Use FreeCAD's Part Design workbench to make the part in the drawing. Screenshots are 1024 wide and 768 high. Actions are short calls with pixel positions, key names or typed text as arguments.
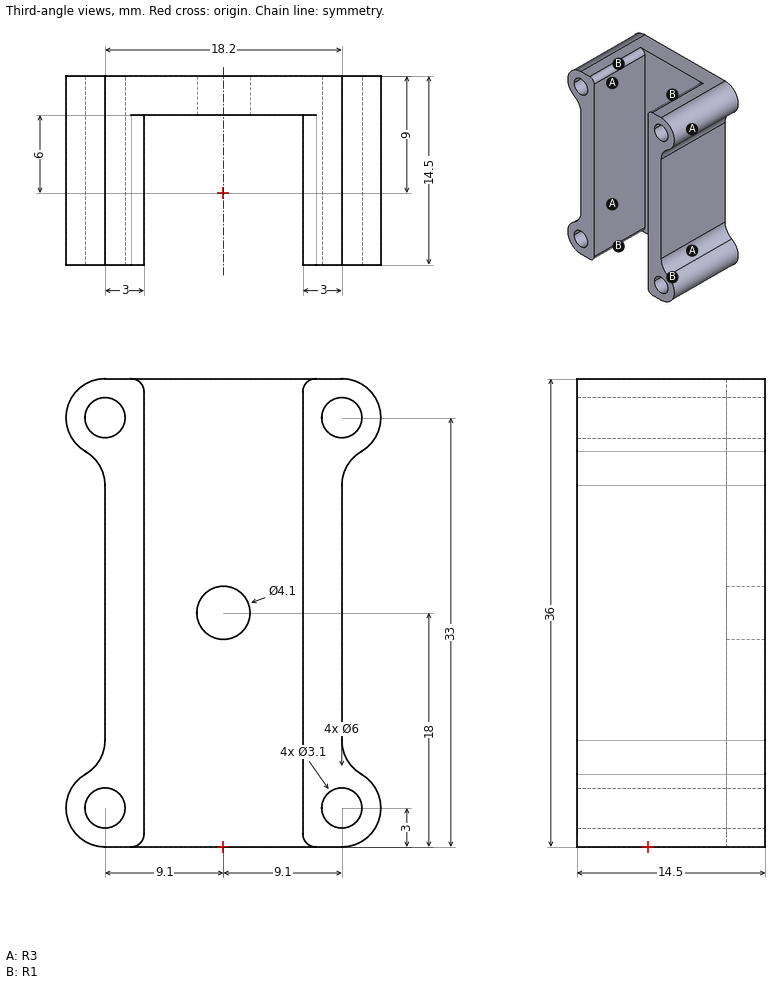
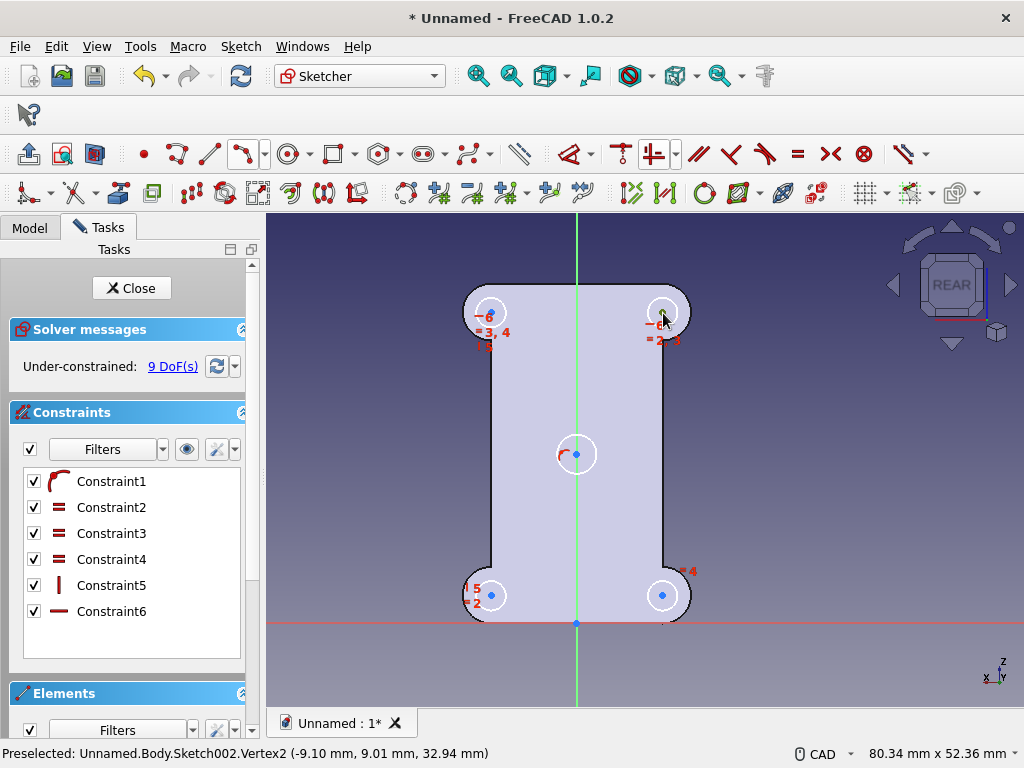
click(663, 596)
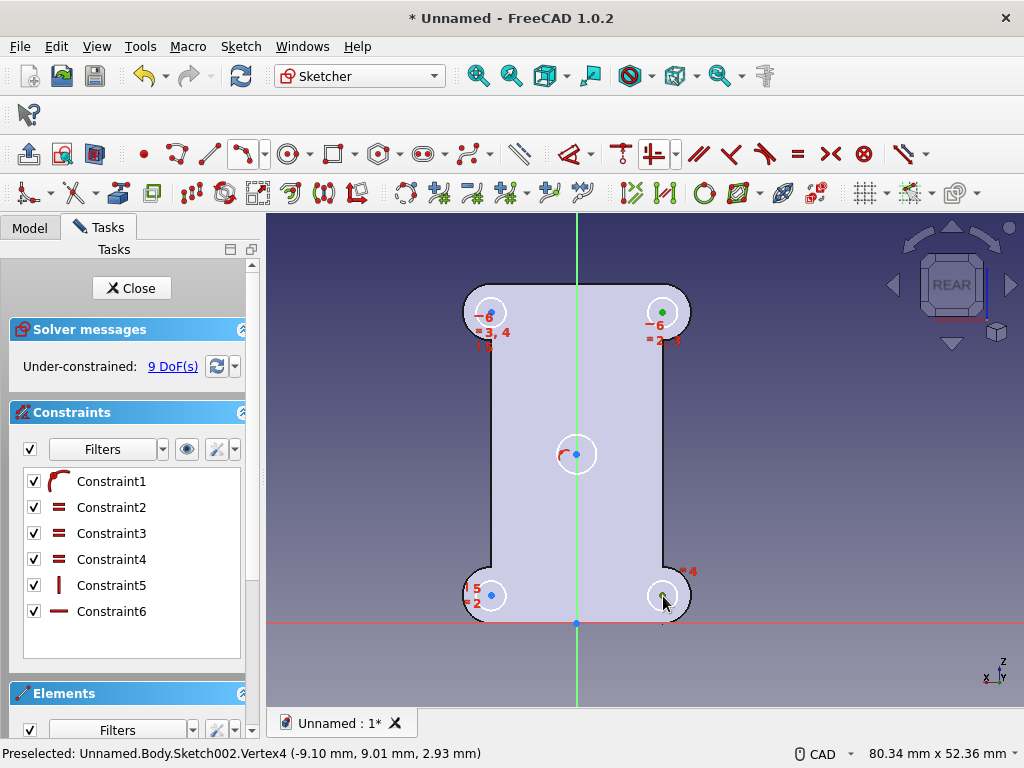
key(v)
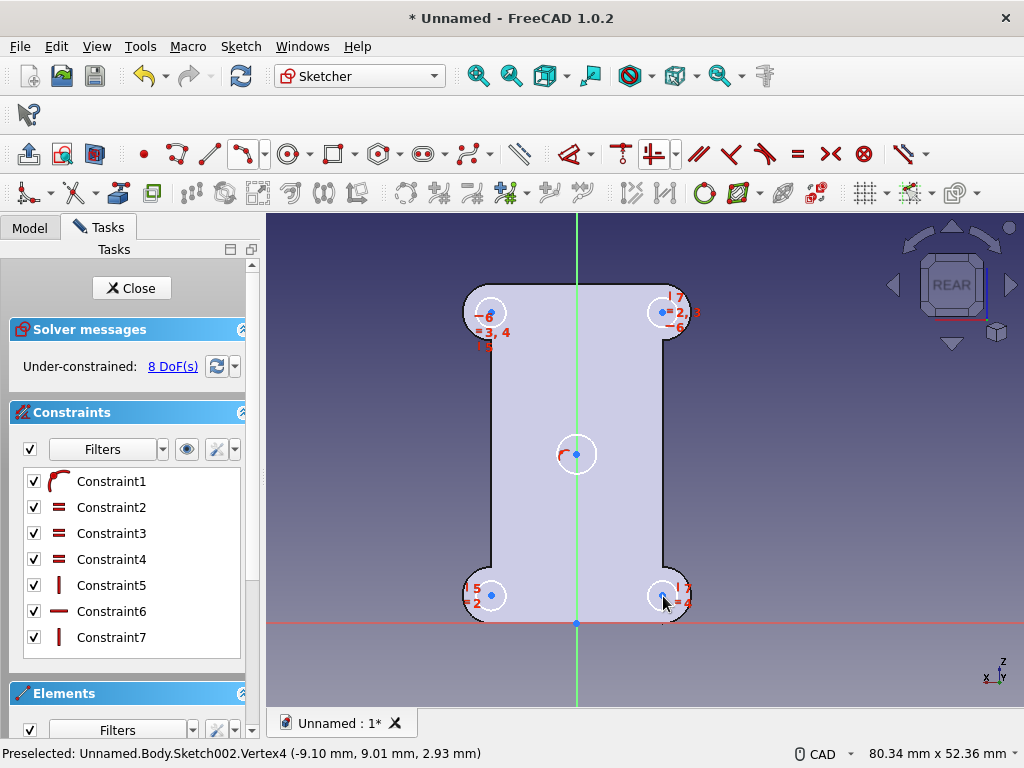
click(491, 596)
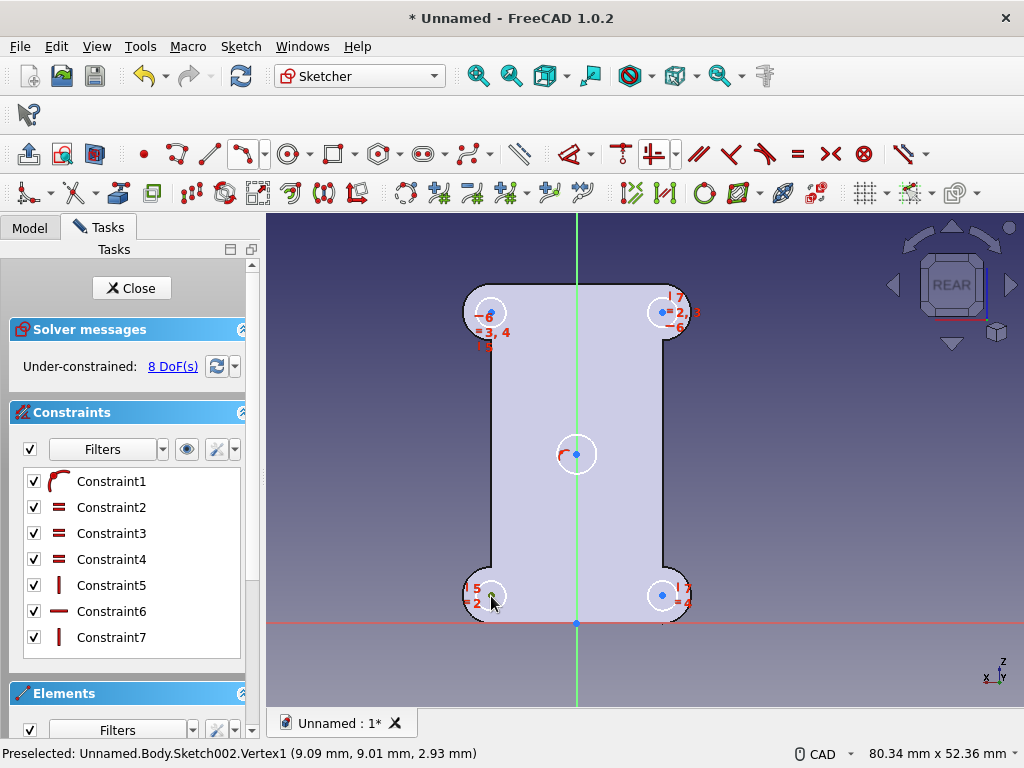
click(663, 596)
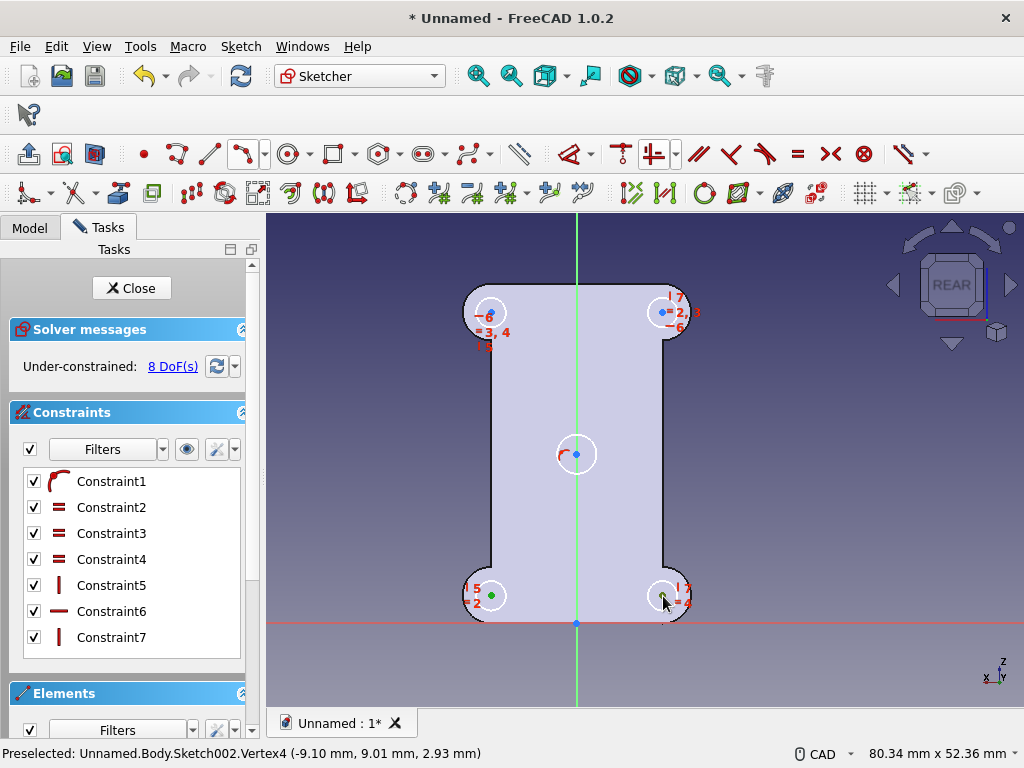
key(h)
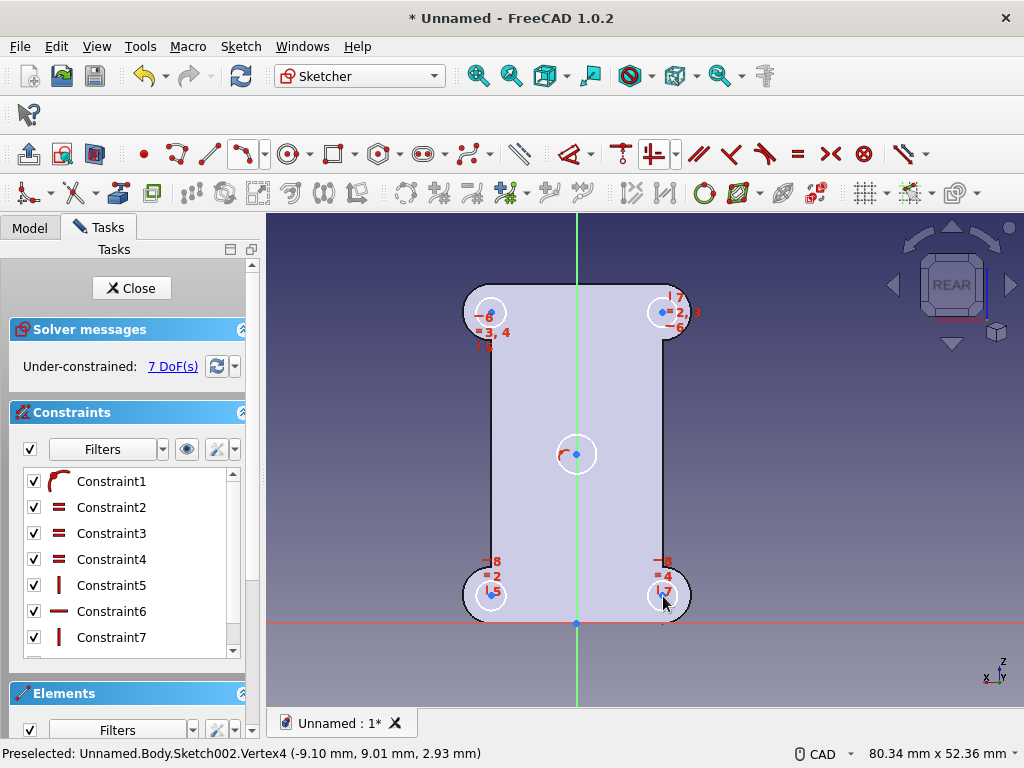
click(568, 154)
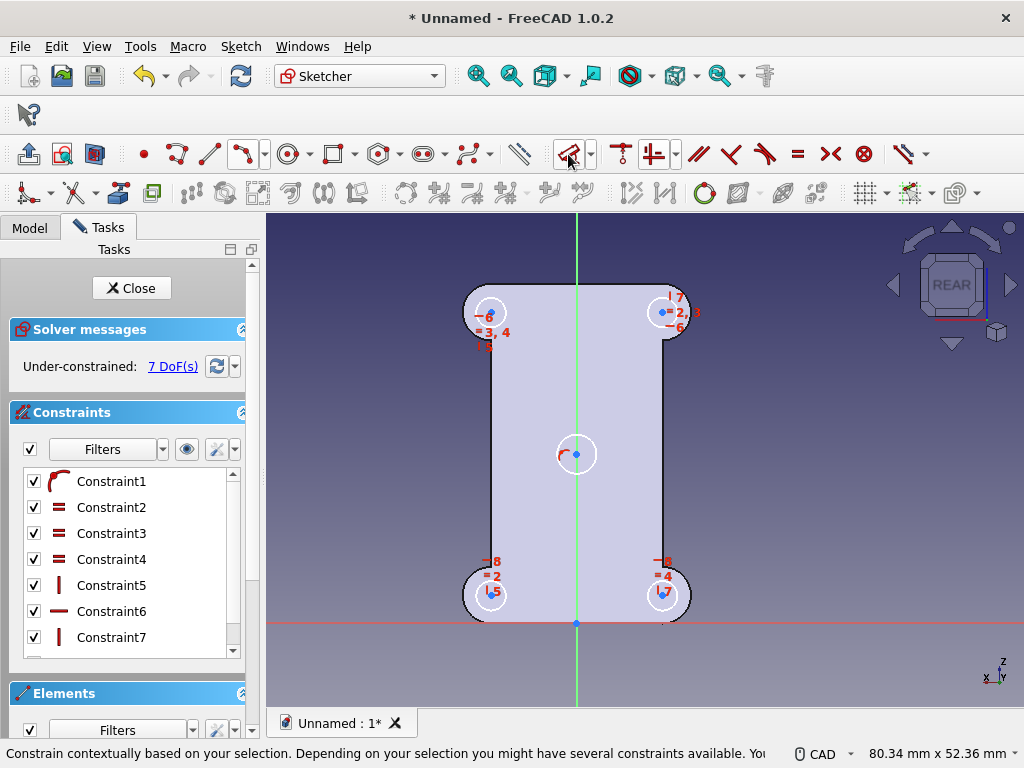
scroll(501, 585, up, 2)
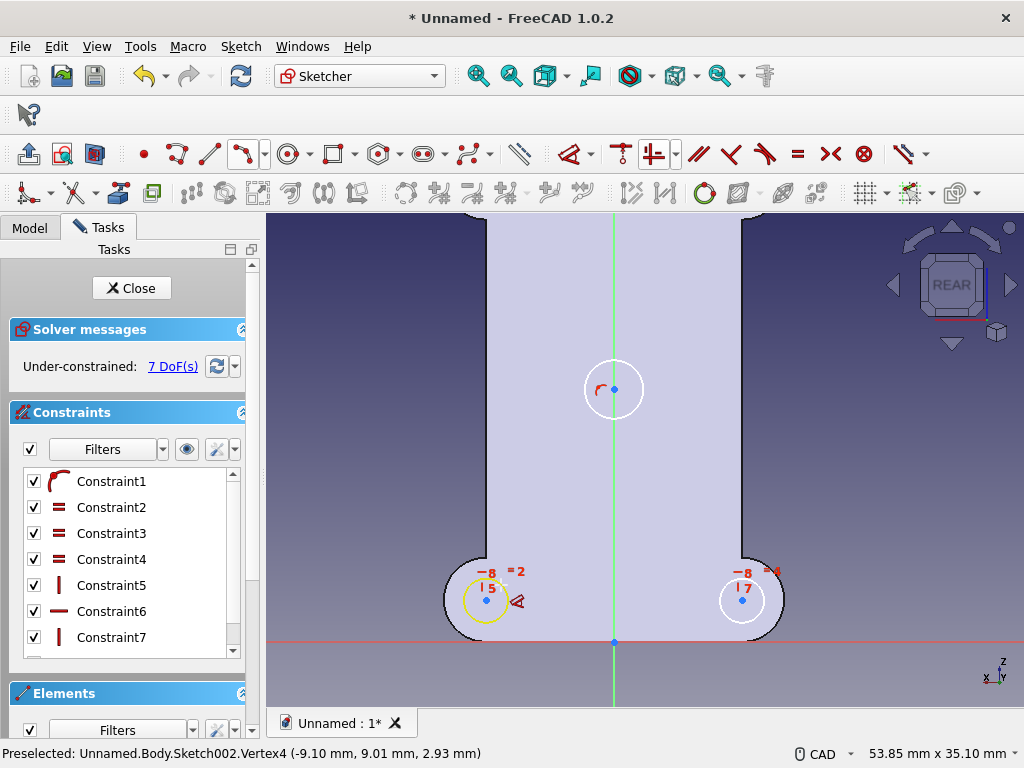
click(502, 585)
click(525, 563)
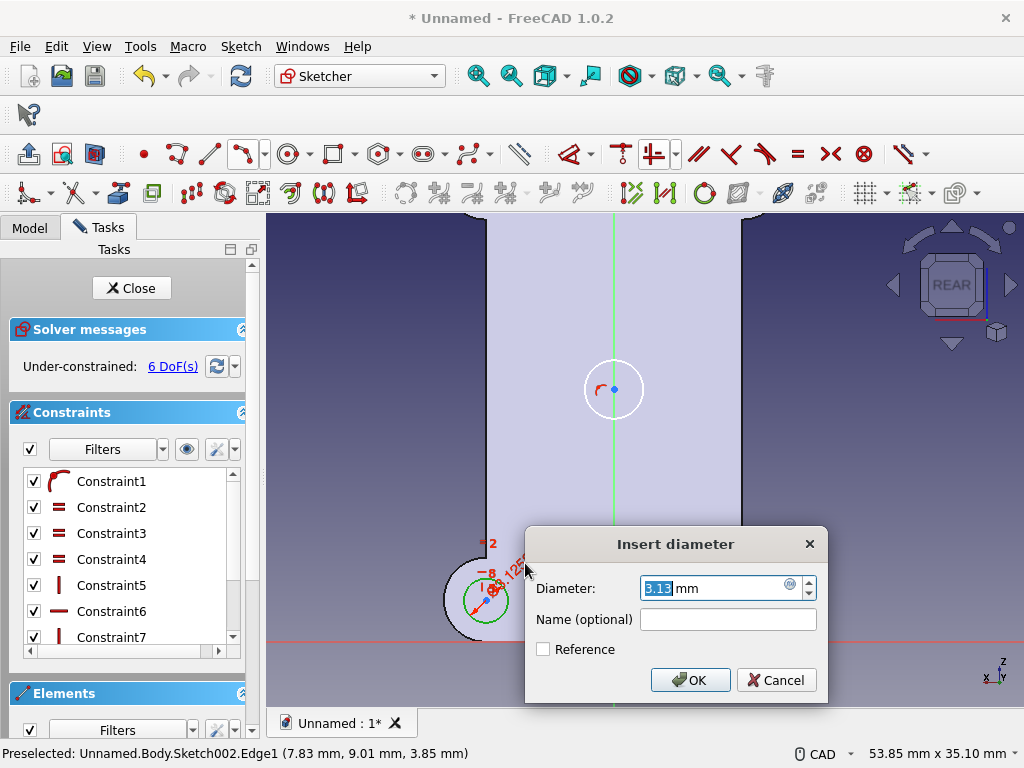
text(3.1)
key(Return)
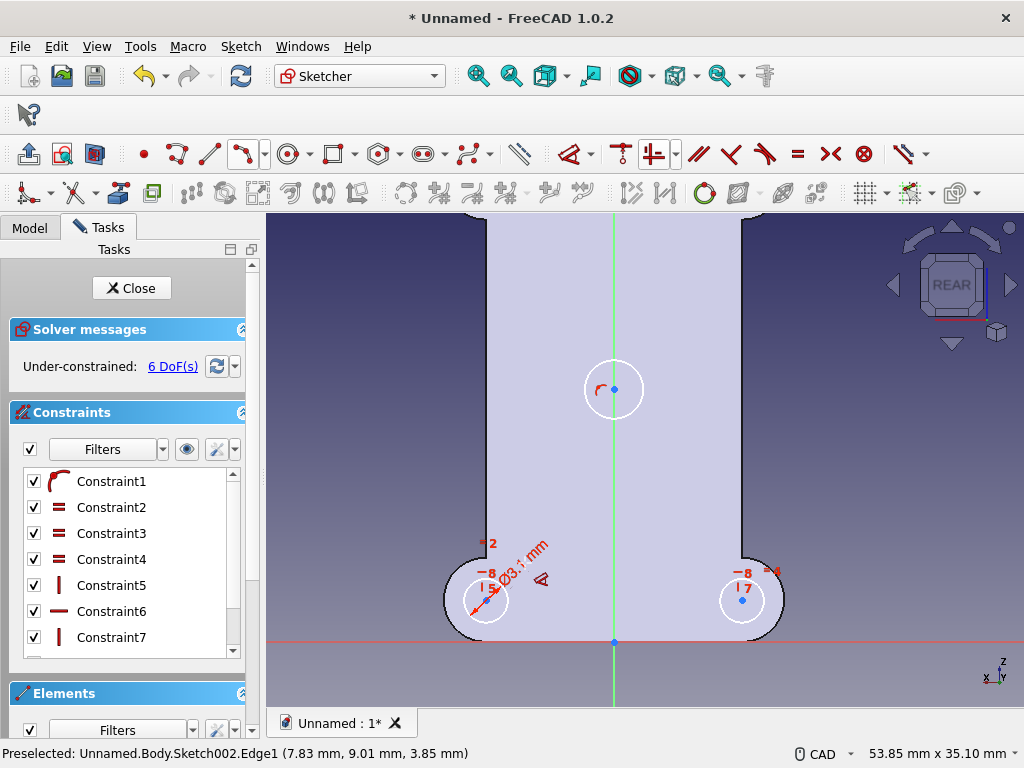
click(635, 369)
click(658, 347)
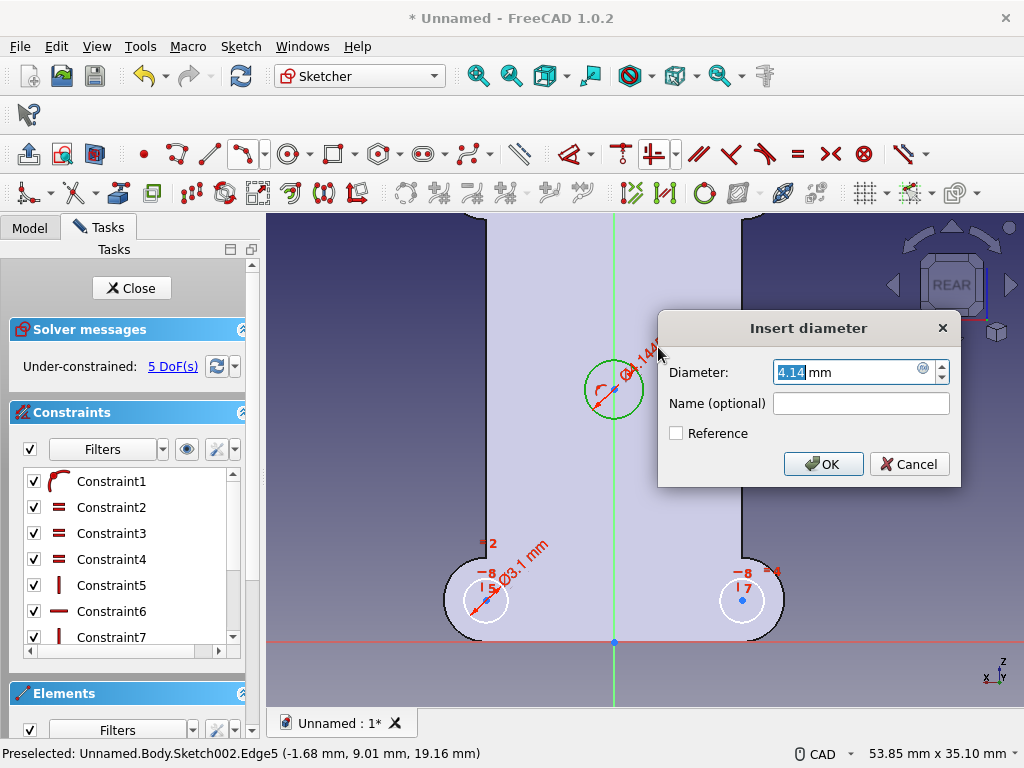
text(4.1)
key(Return)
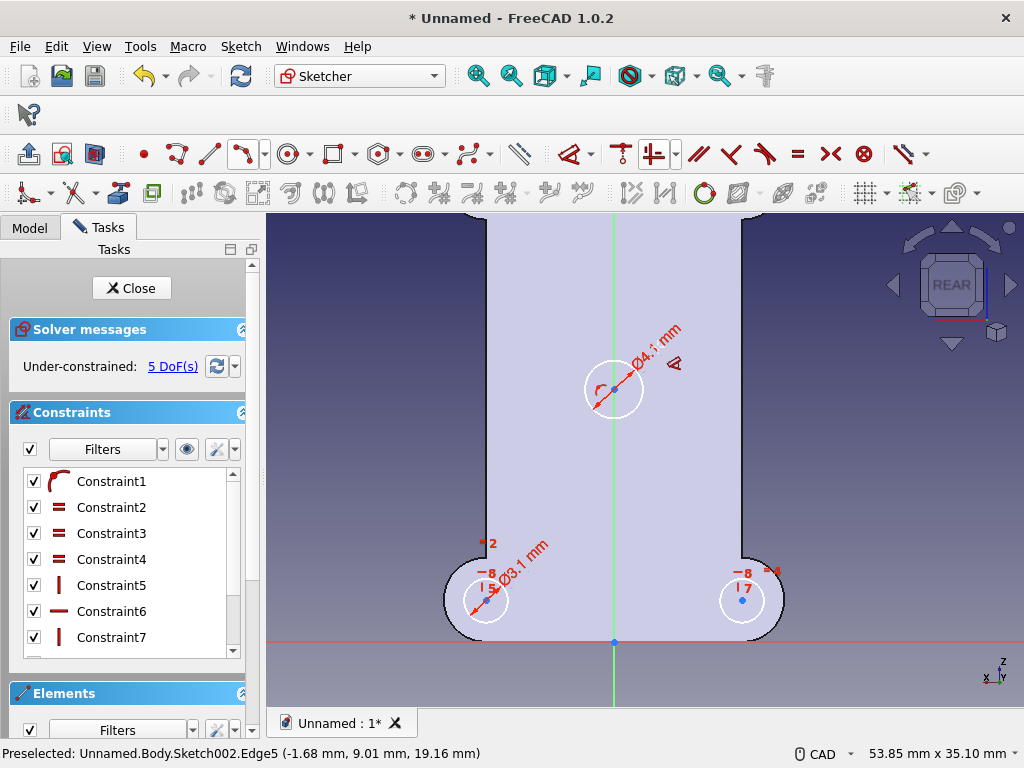
click(486, 601)
click(452, 621)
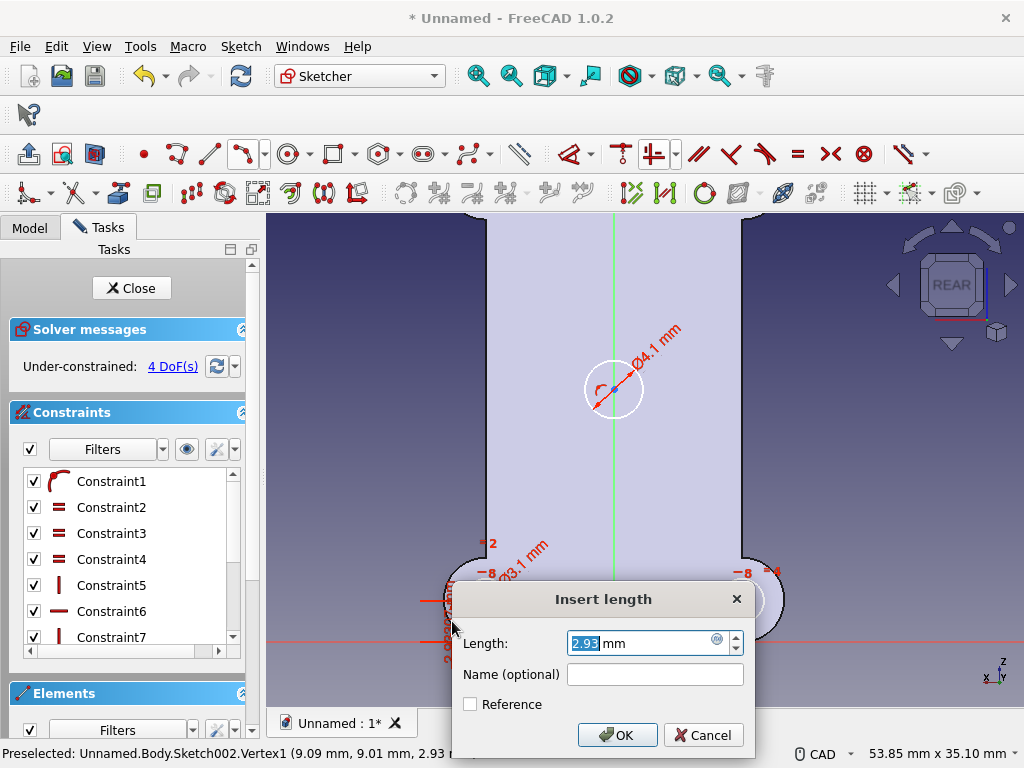
text(3)
key(Return)